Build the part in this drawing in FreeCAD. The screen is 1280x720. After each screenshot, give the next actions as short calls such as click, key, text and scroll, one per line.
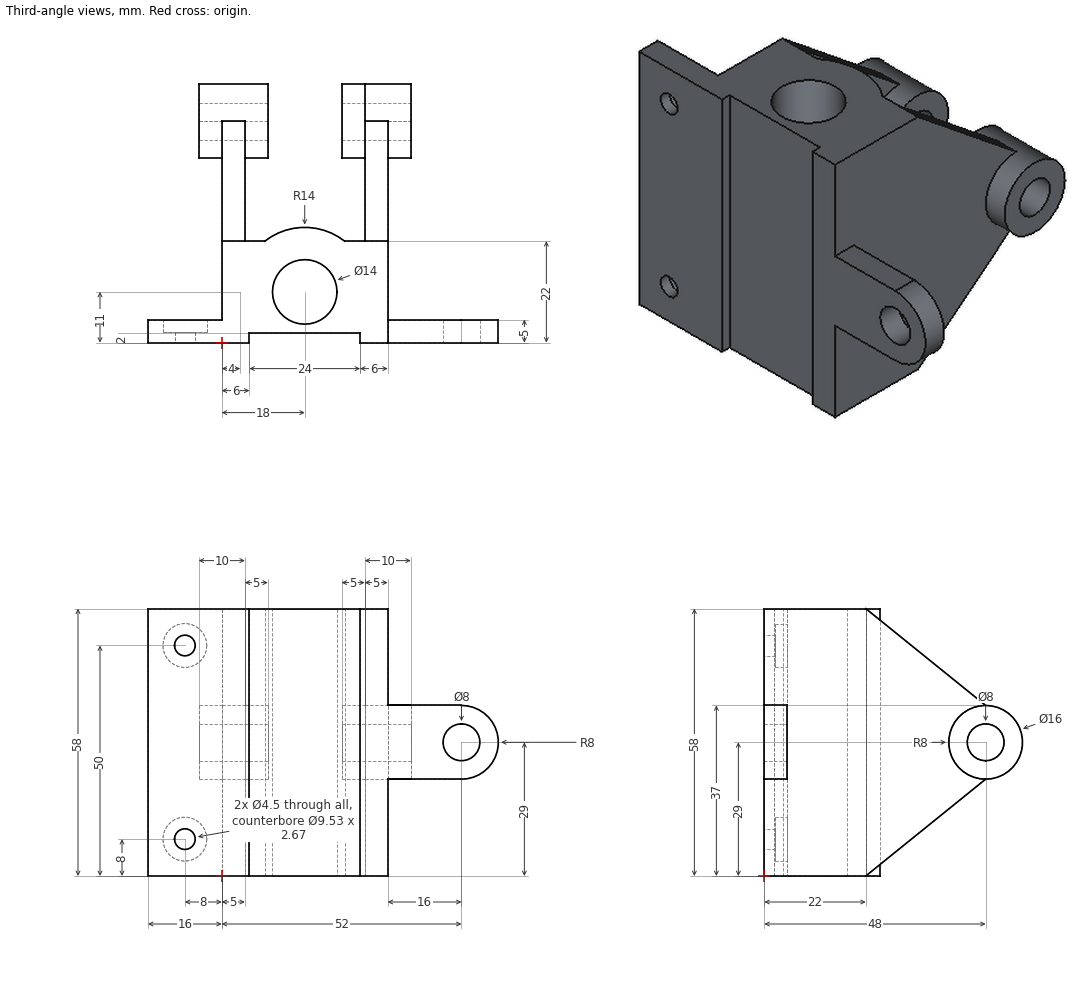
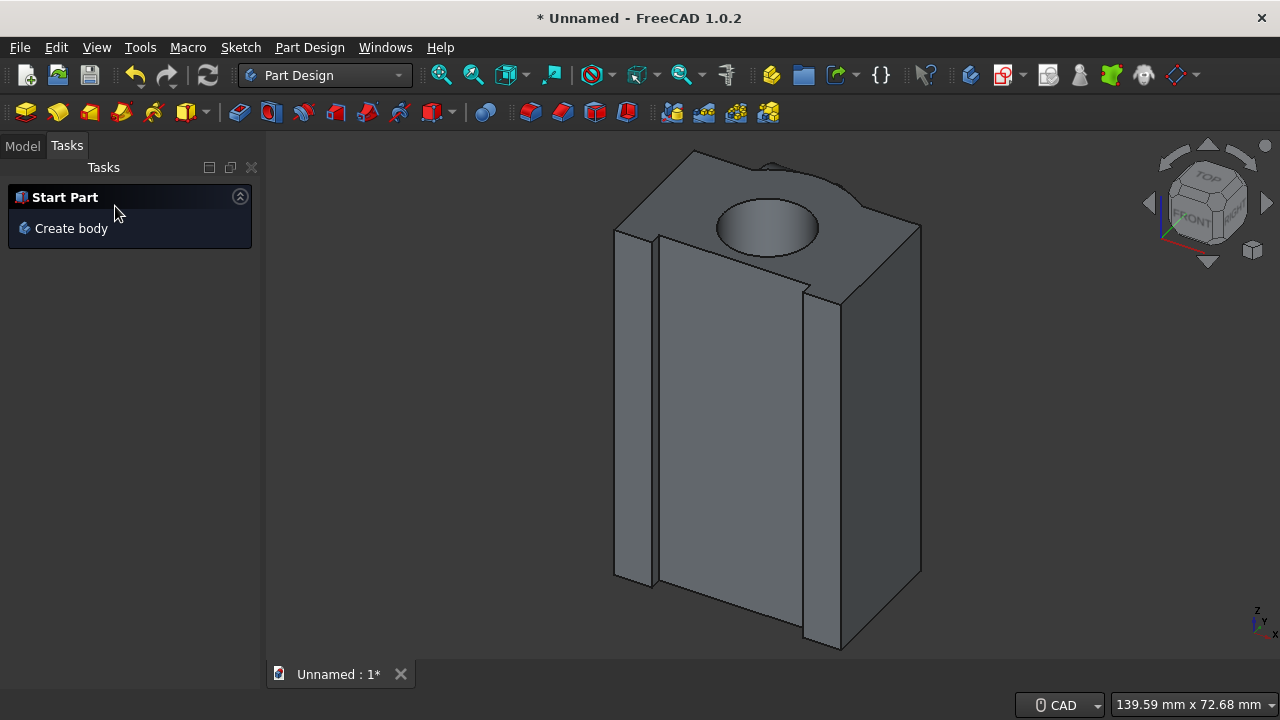
key(v)
key(f)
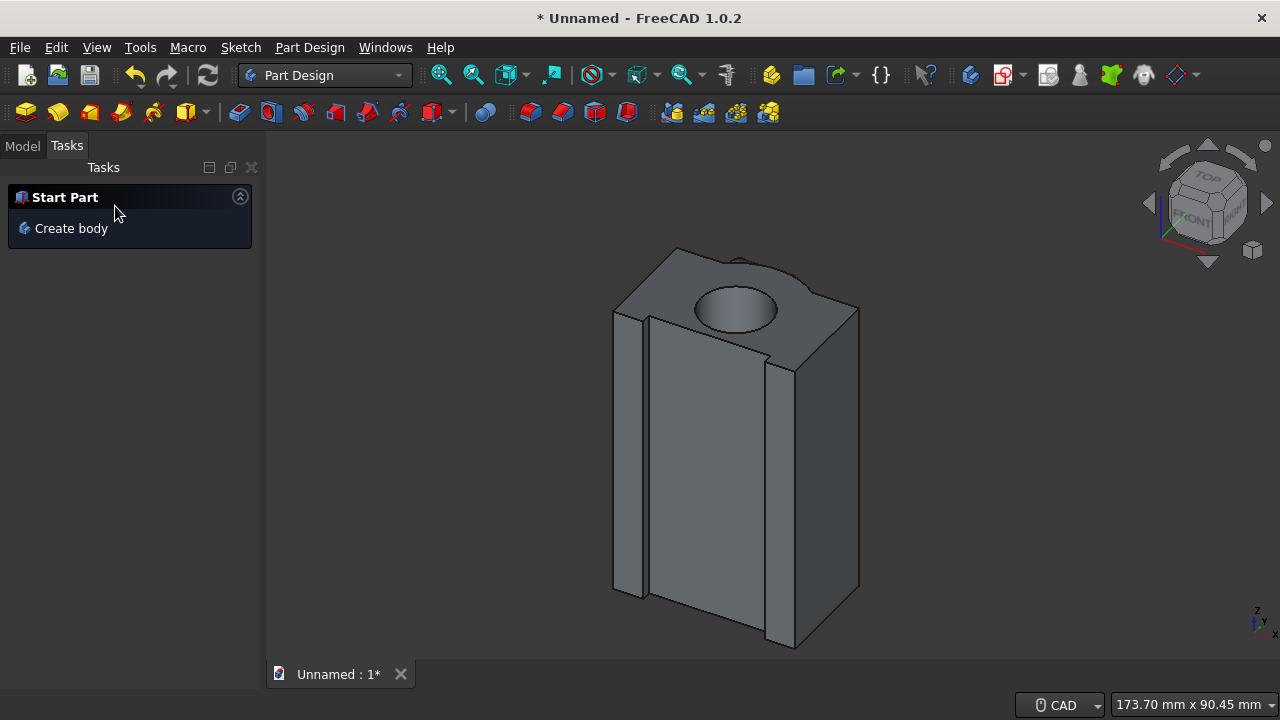
click(23, 145)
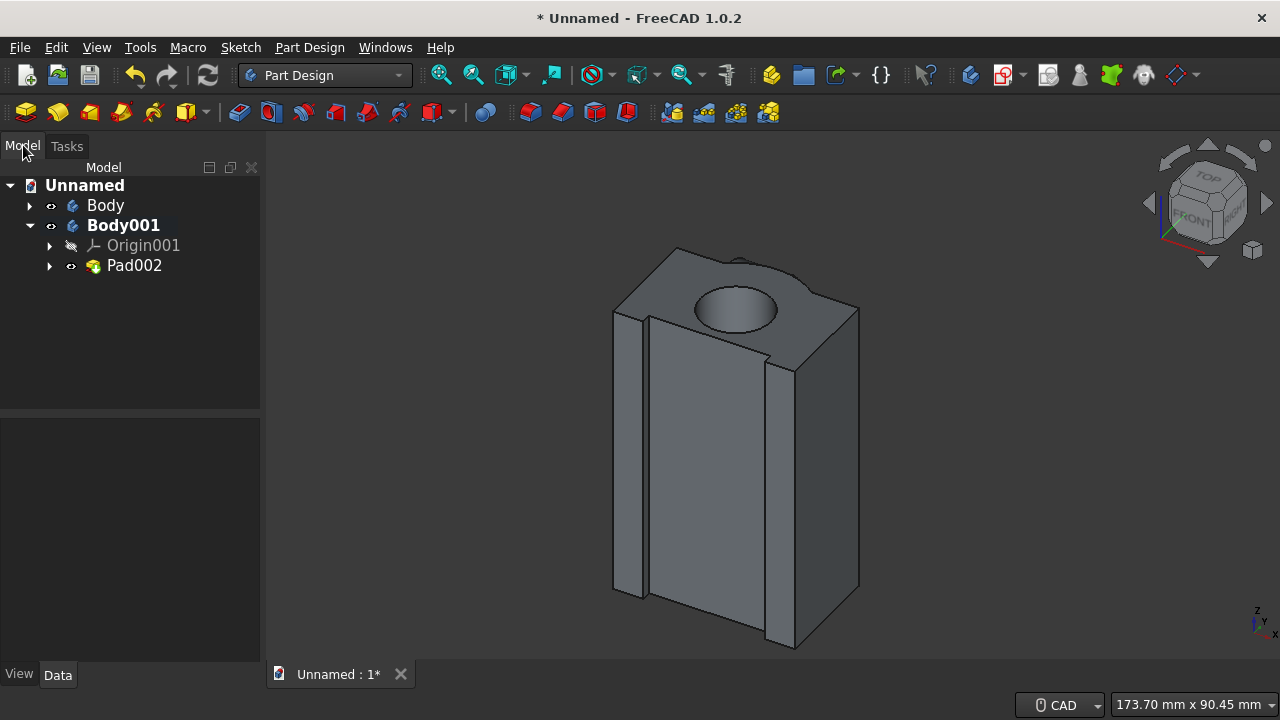
double_click(96, 206)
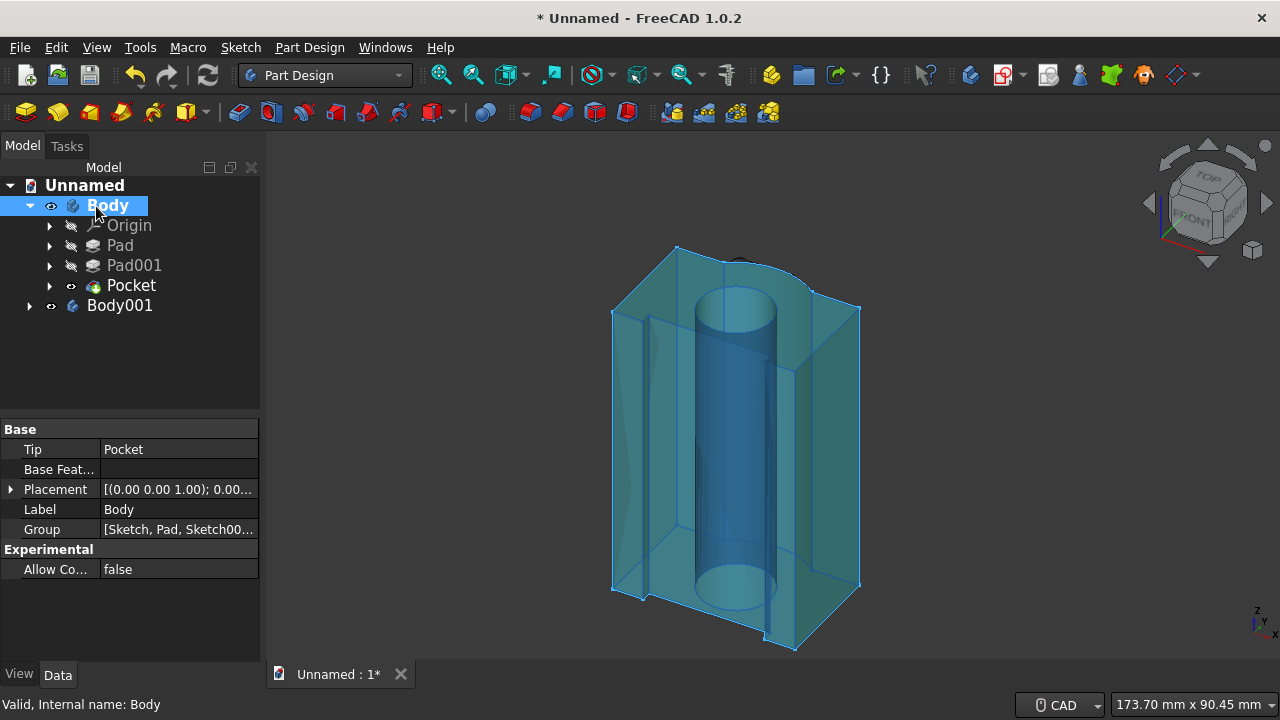
click(96, 206)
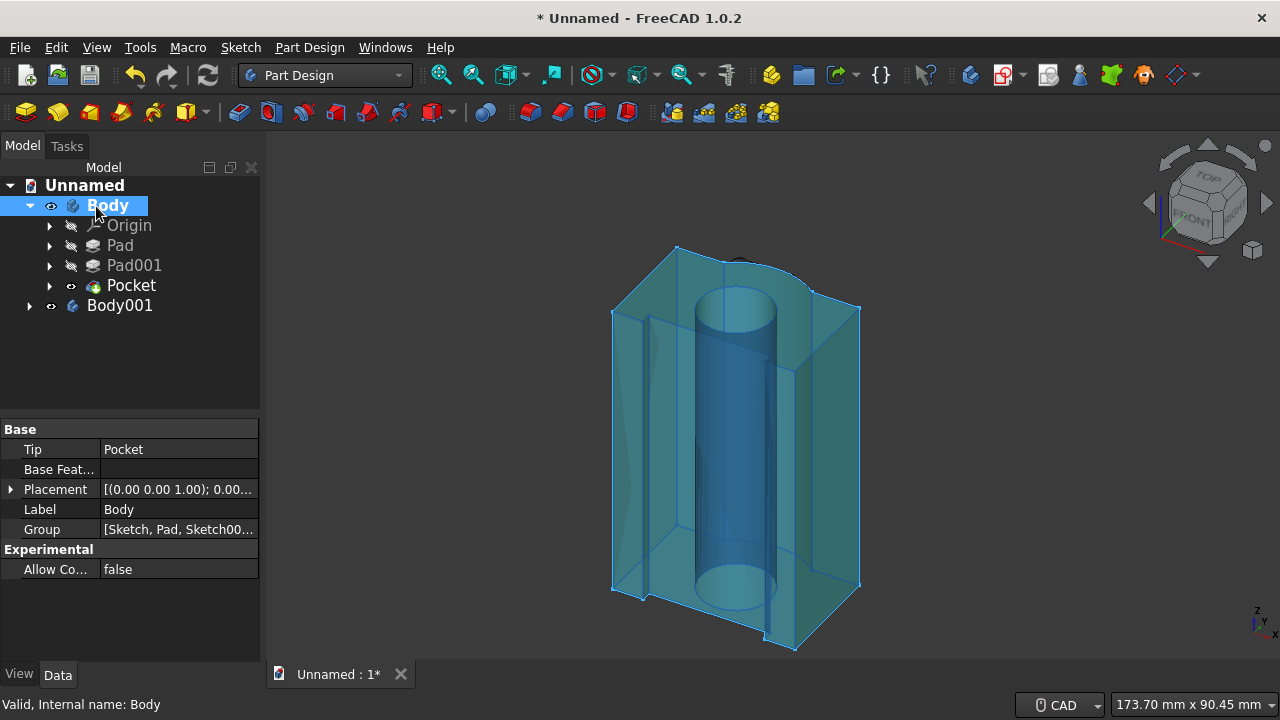
click(146, 569)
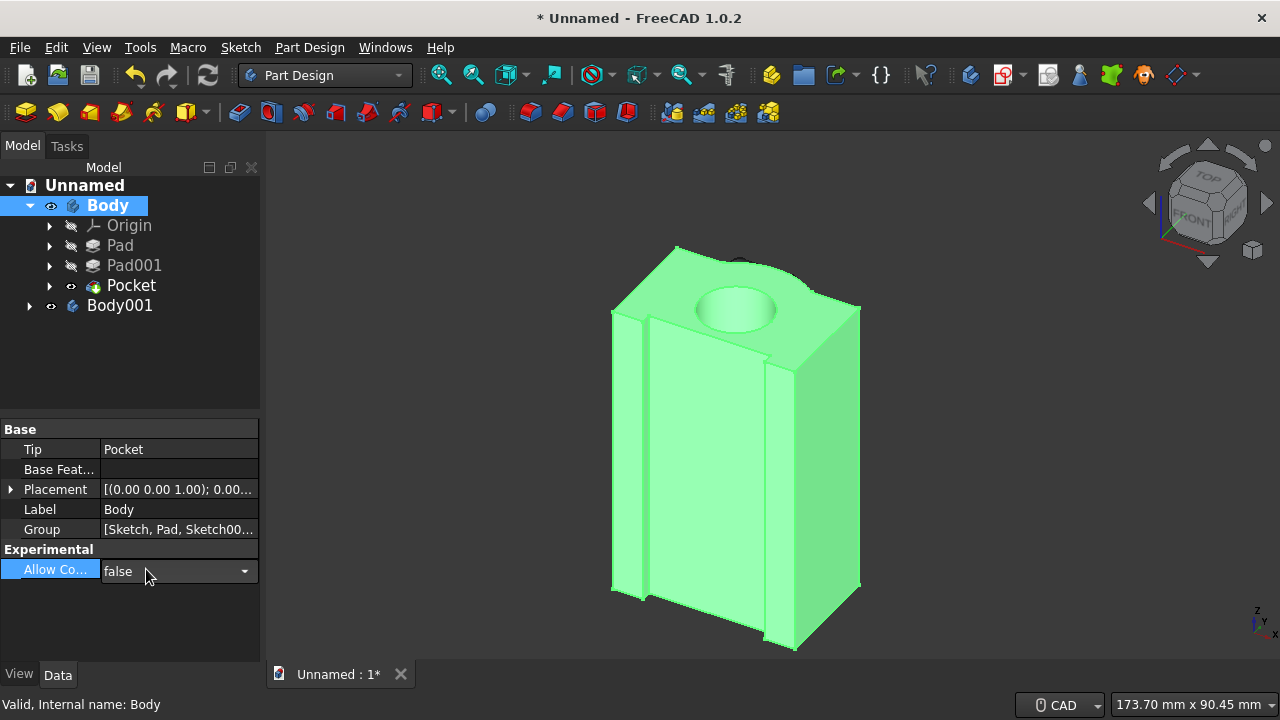
click(146, 569)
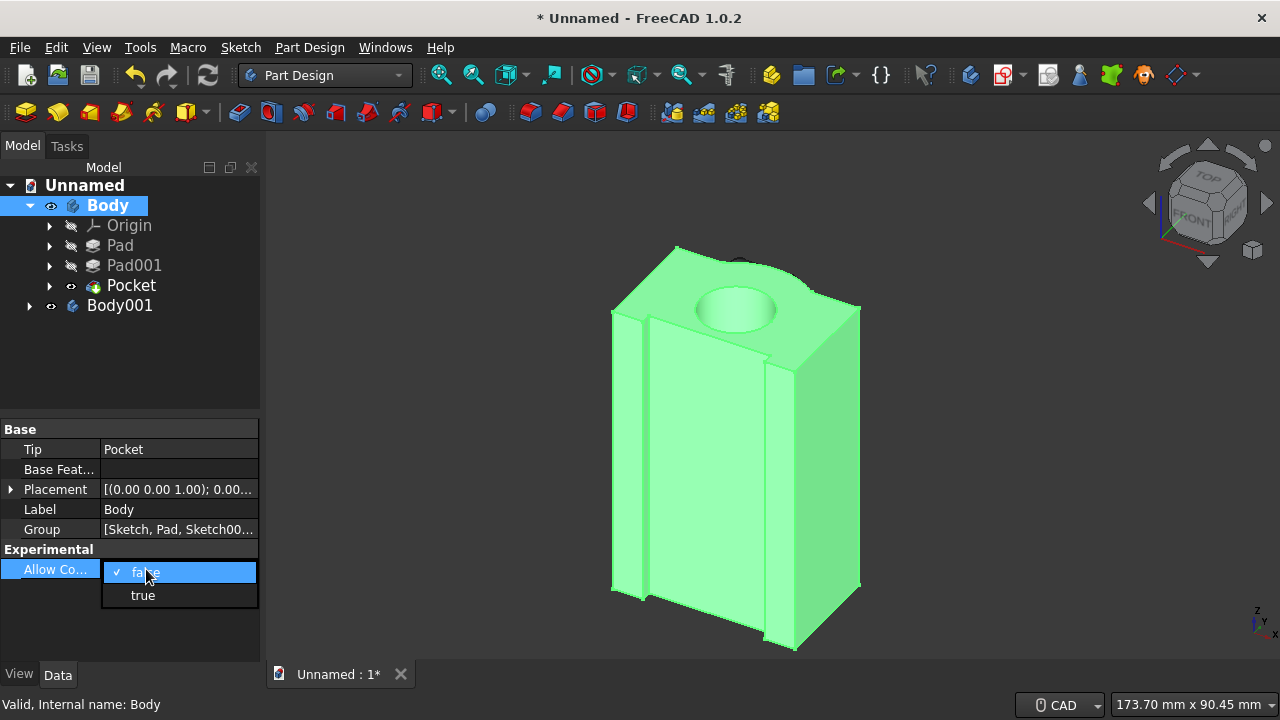
click(179, 596)
key(Return)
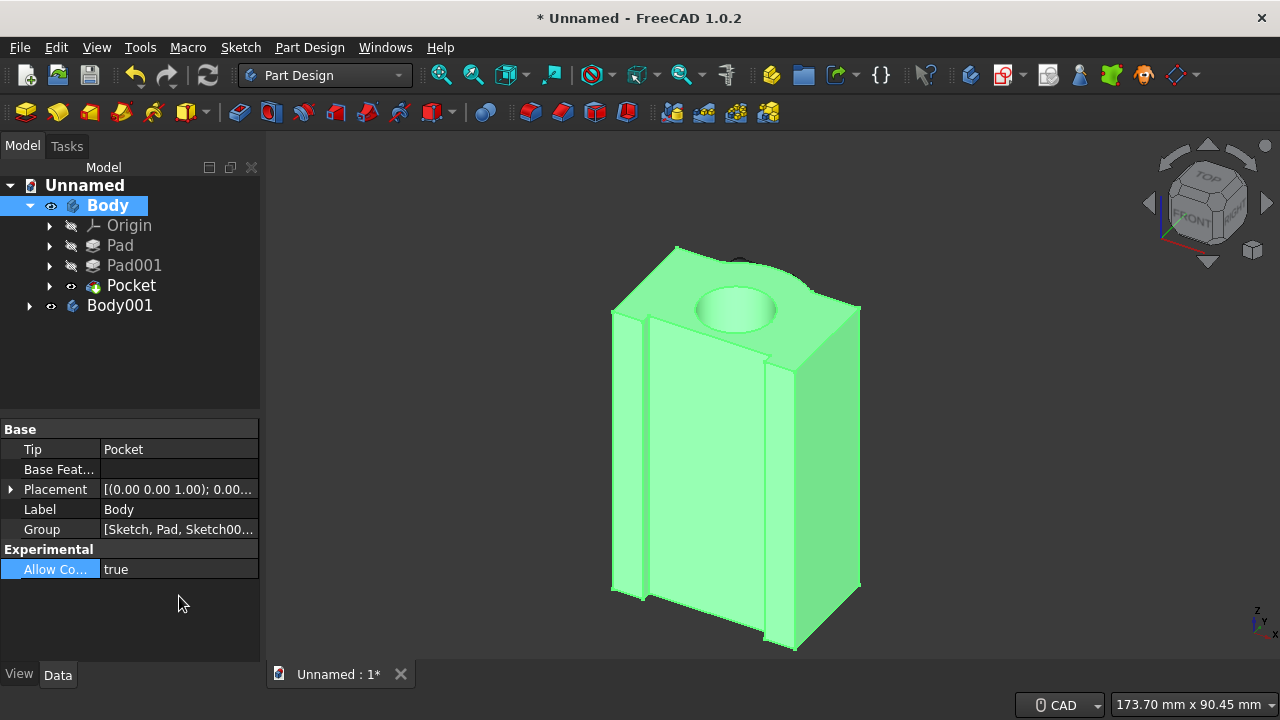
click(96, 306)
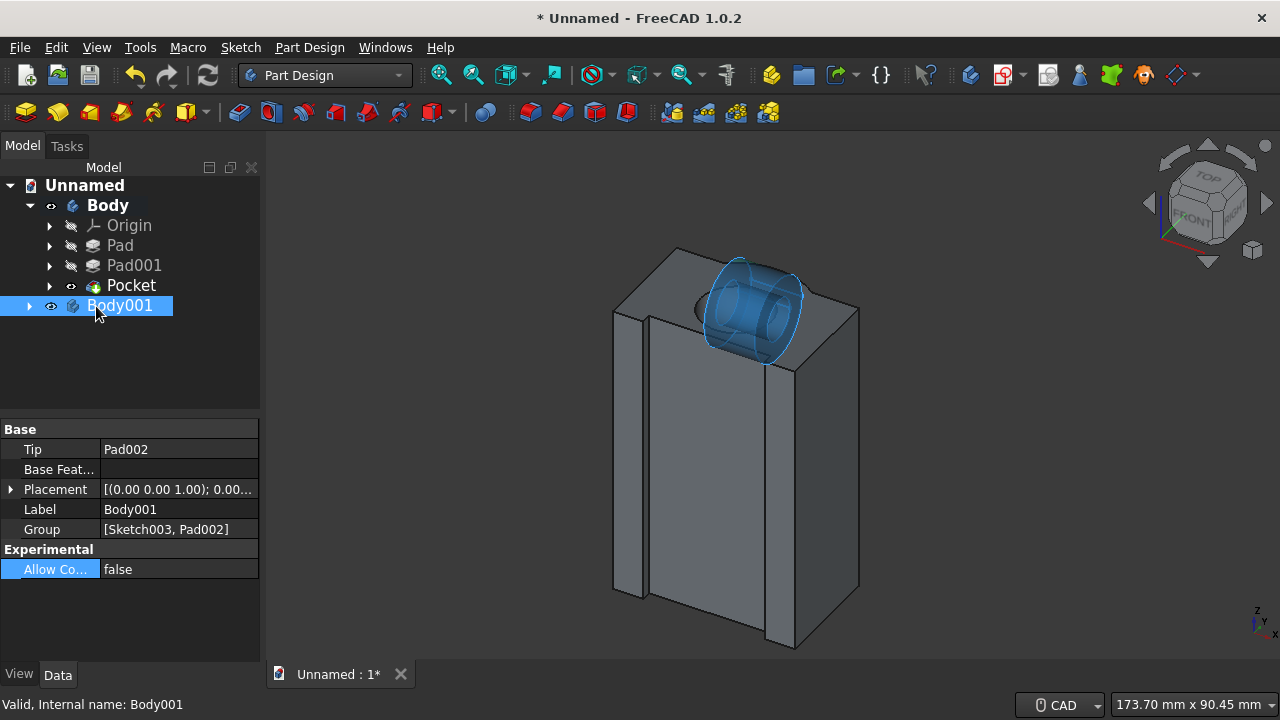
click(486, 112)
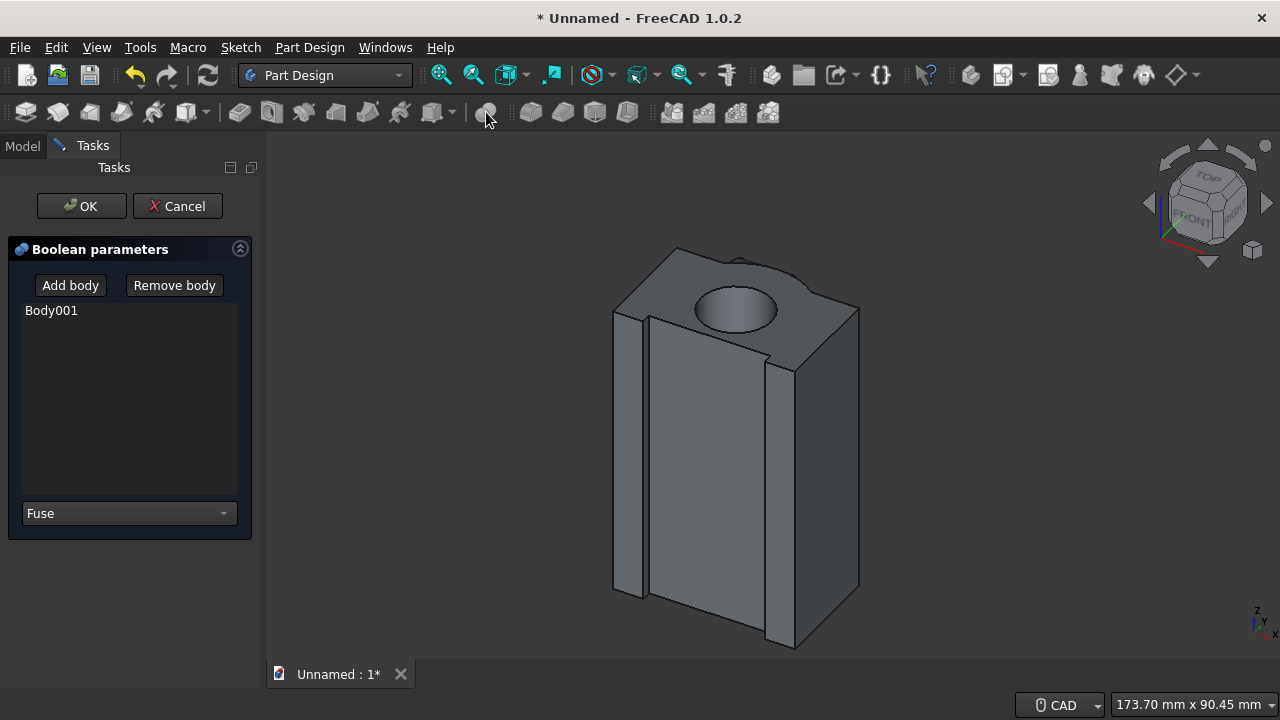
click(82, 206)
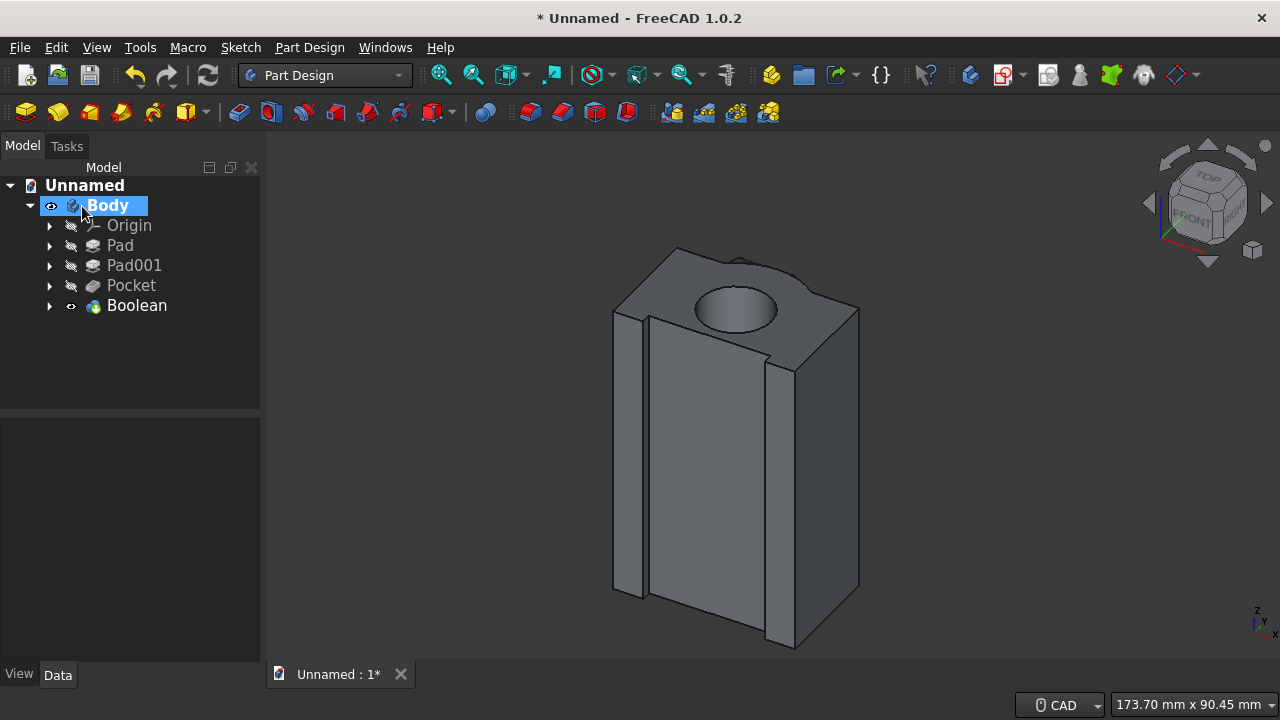
click(1004, 76)